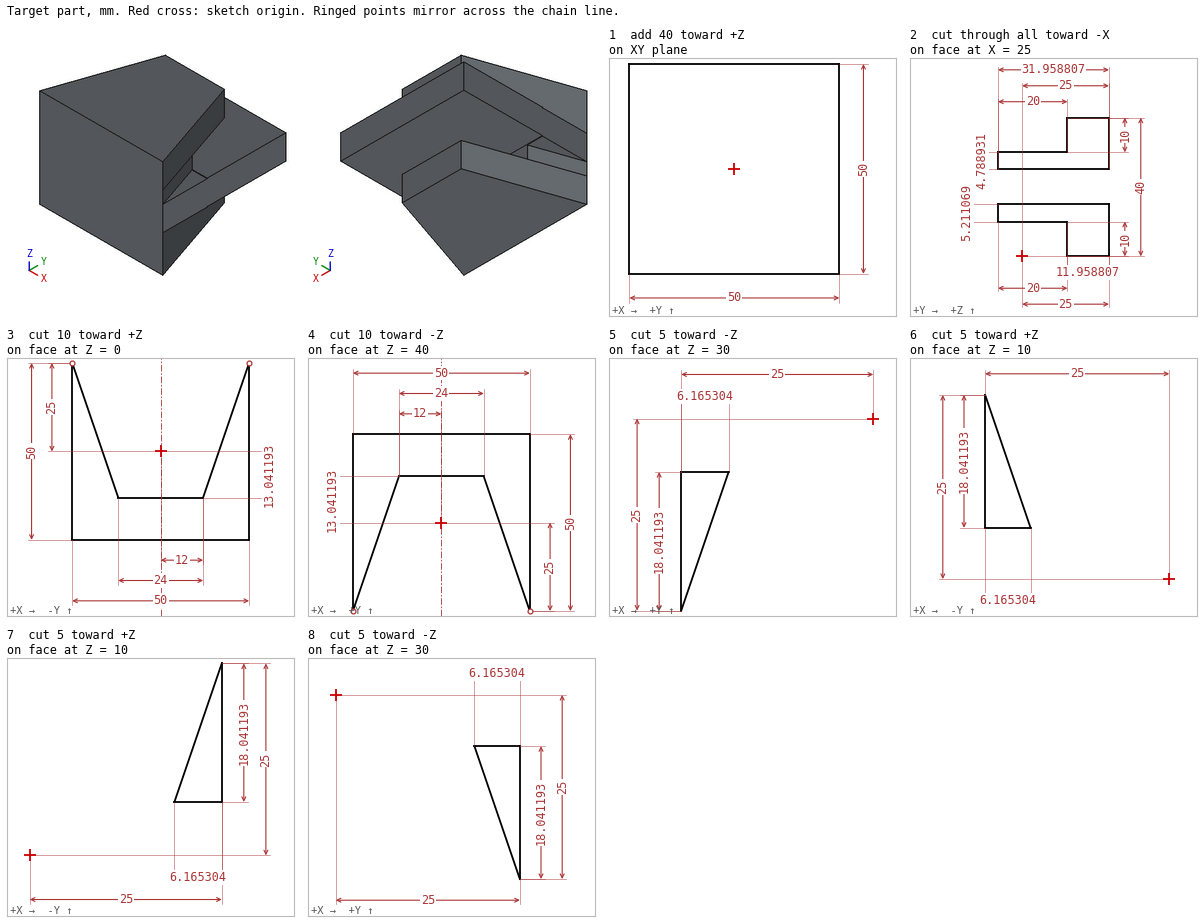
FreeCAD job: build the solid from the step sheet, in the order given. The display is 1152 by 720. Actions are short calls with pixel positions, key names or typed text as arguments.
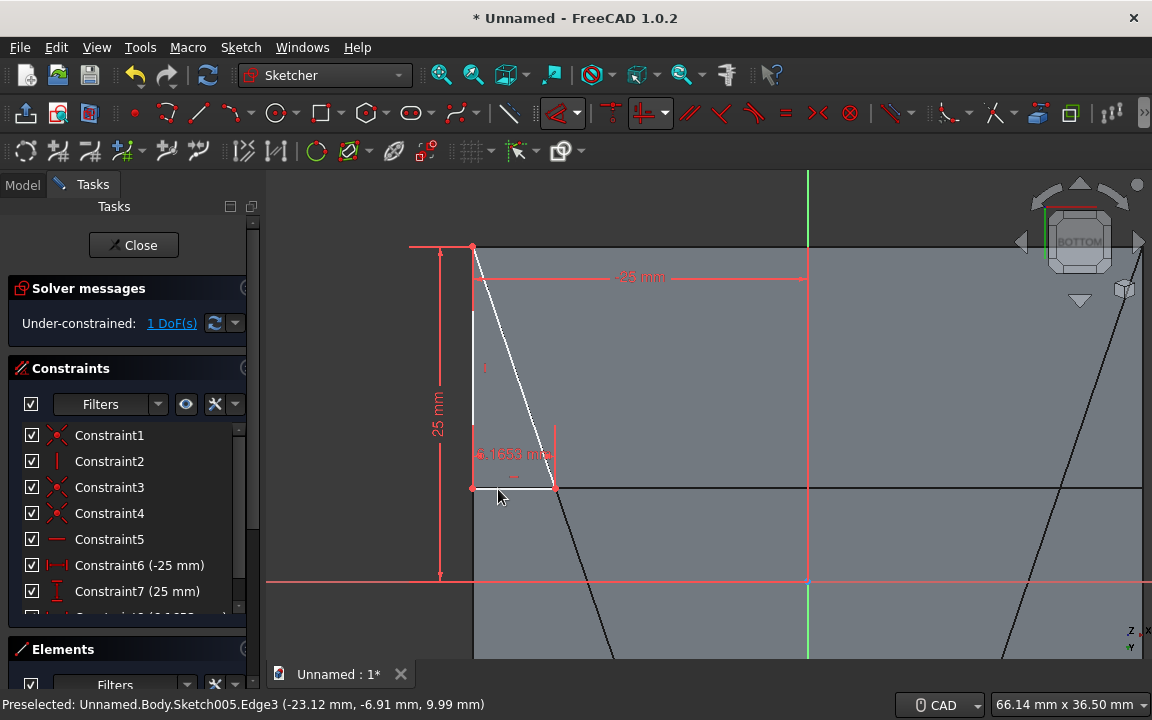
click(473, 319)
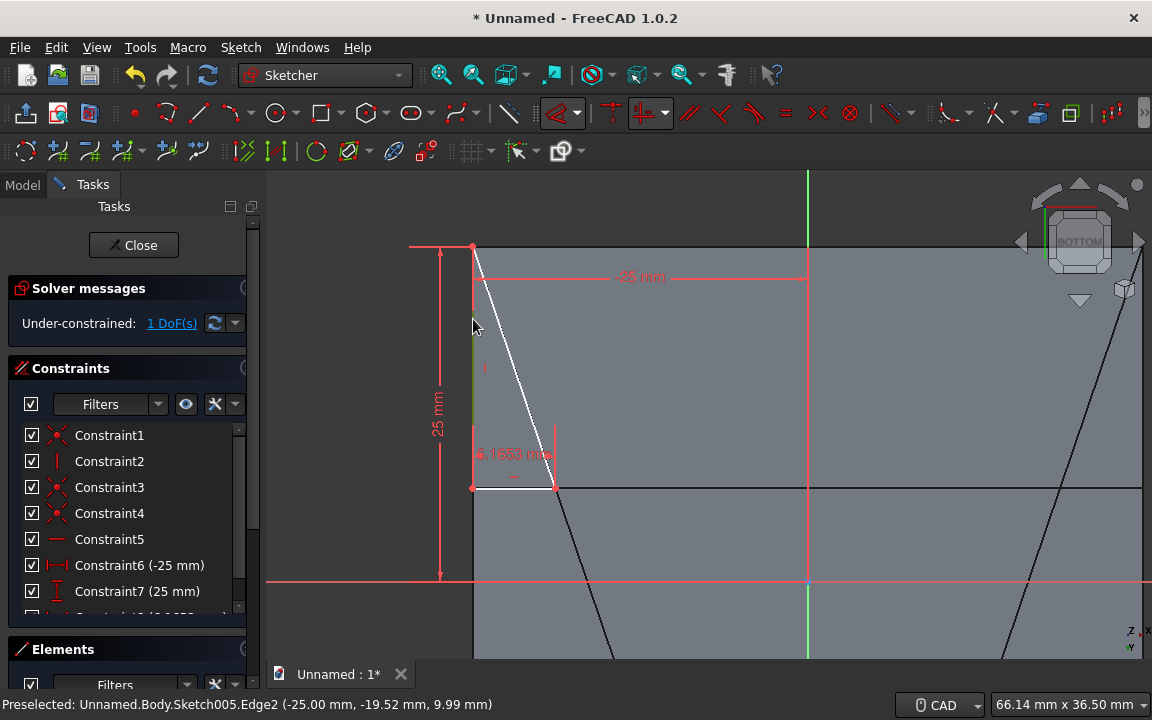
key(i)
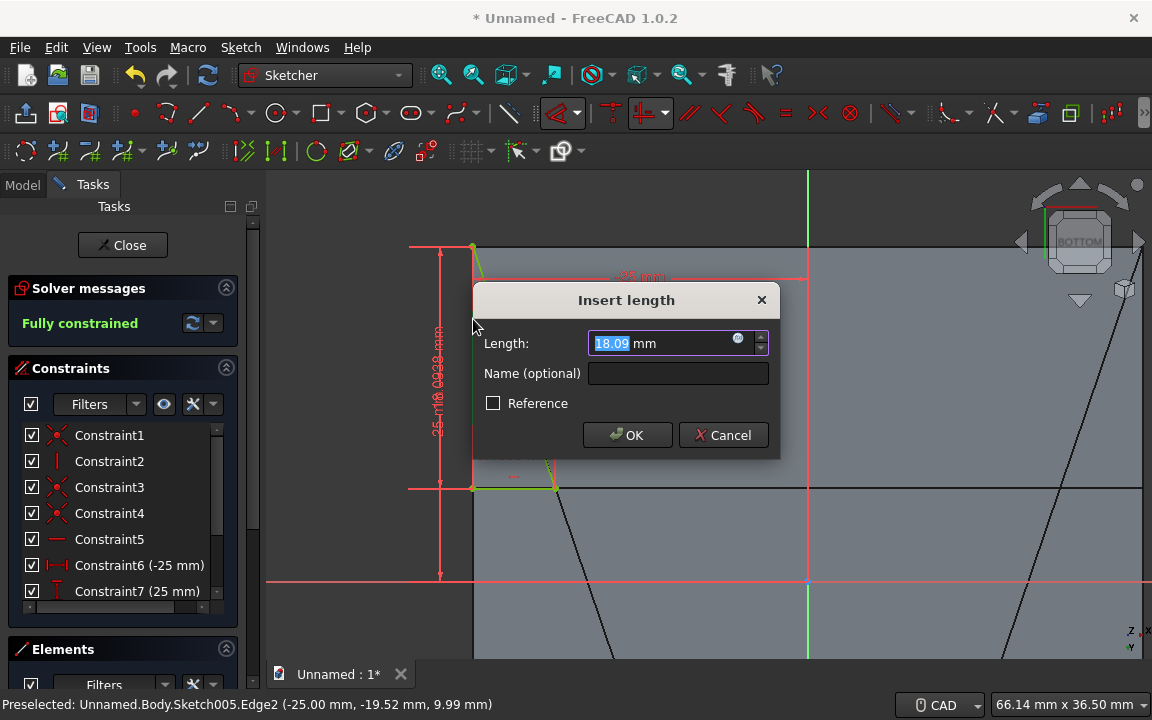
text(18.041193)
key(Return)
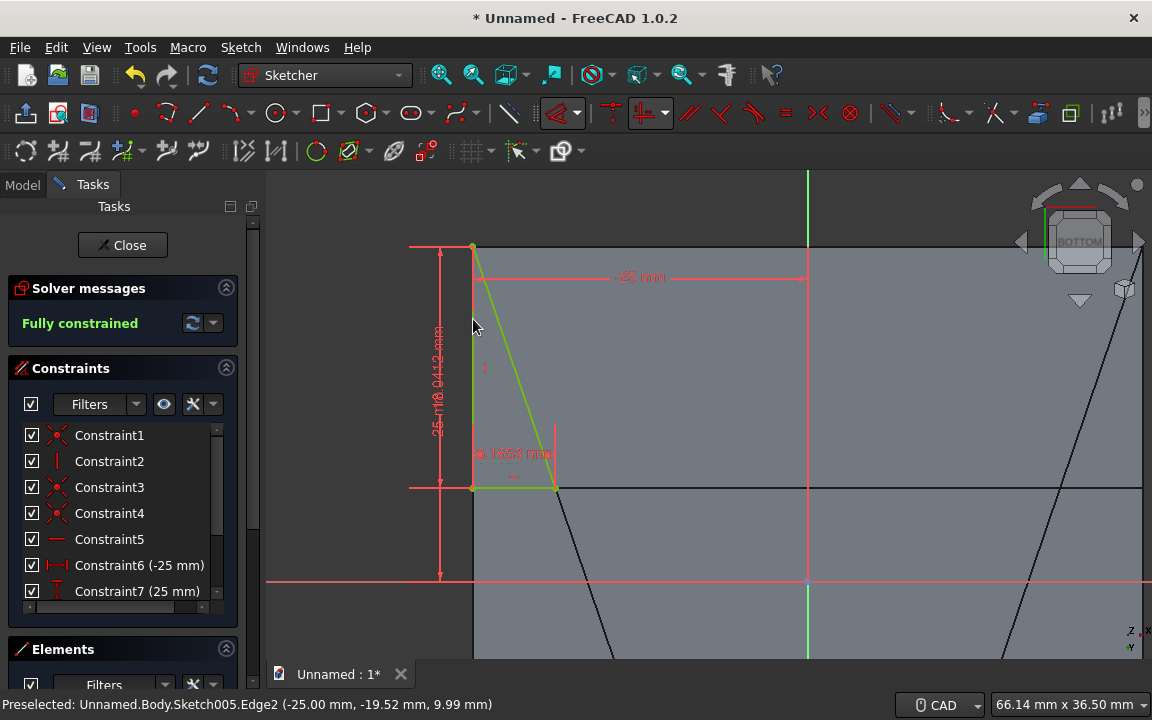
click(123, 245)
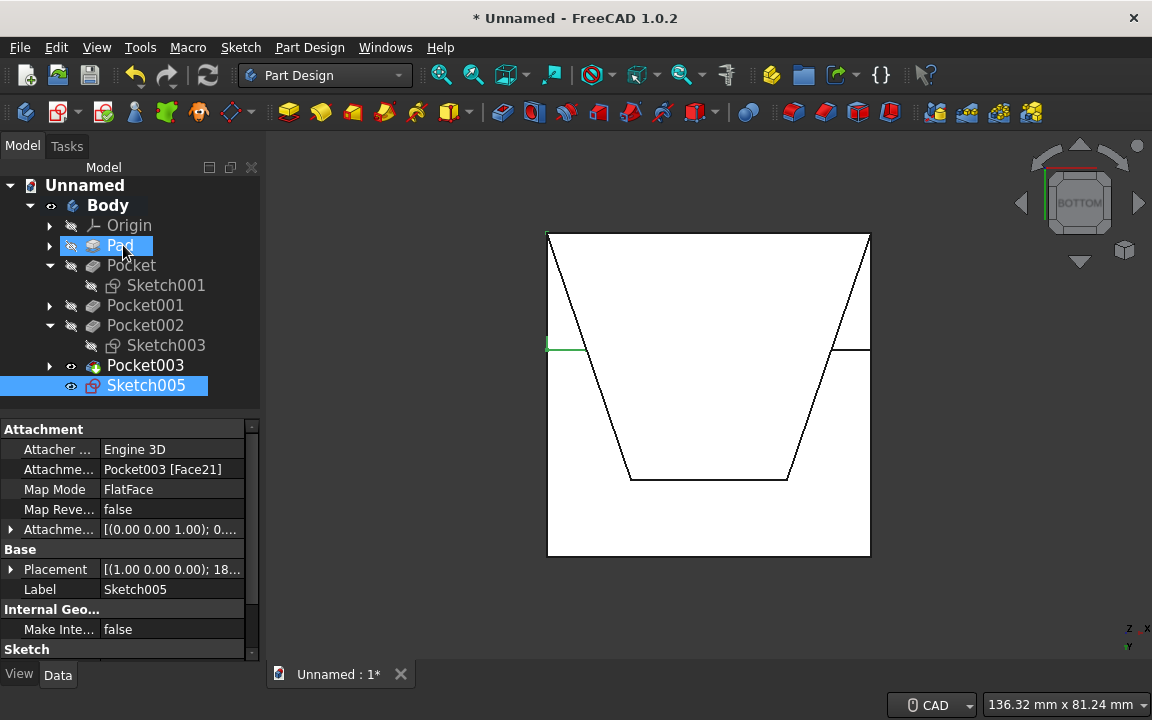
click(504, 112)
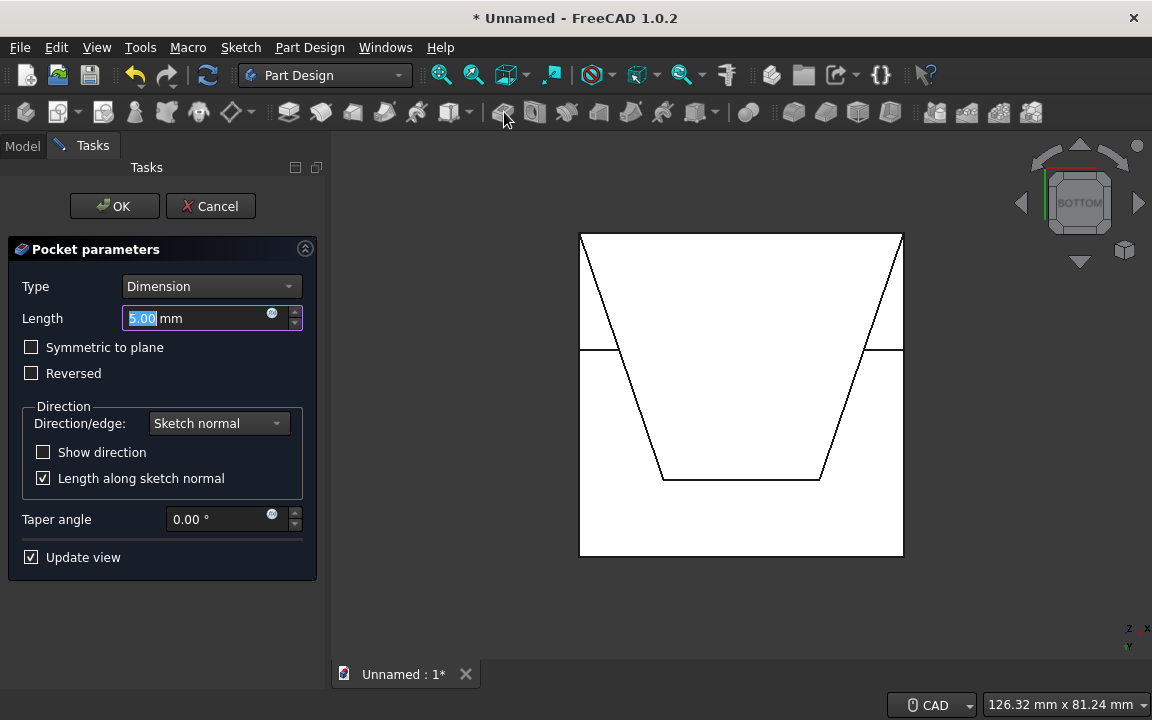
text(5)
key(Tab)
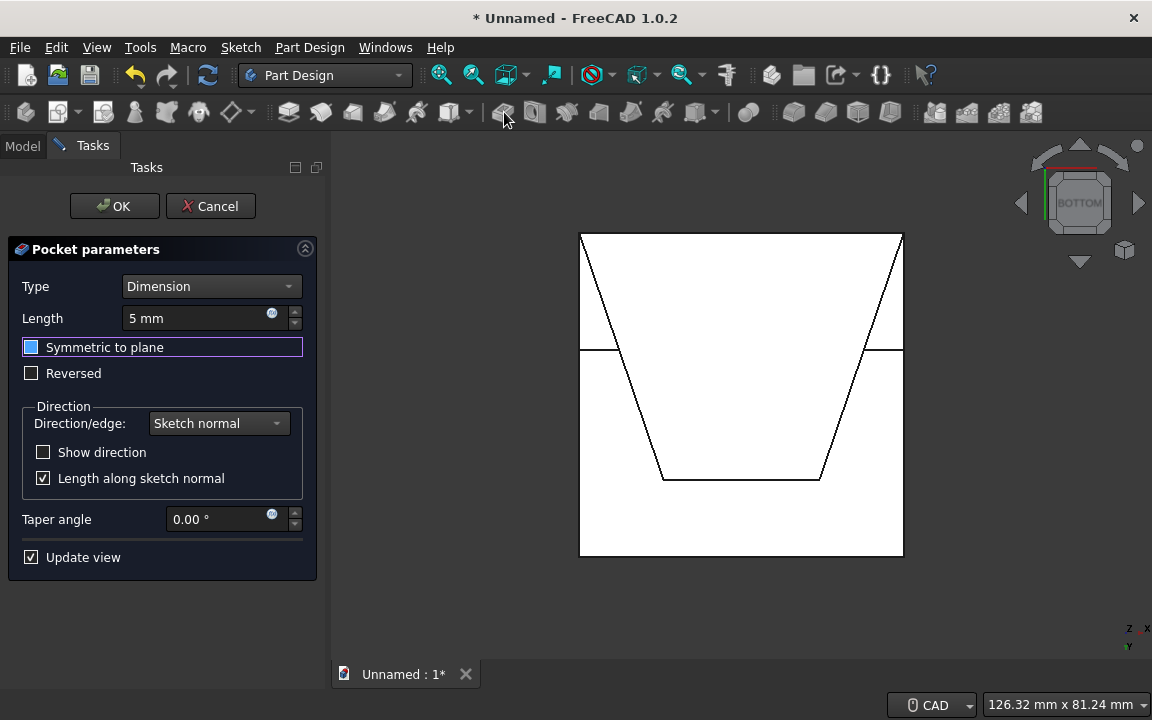
click(115, 206)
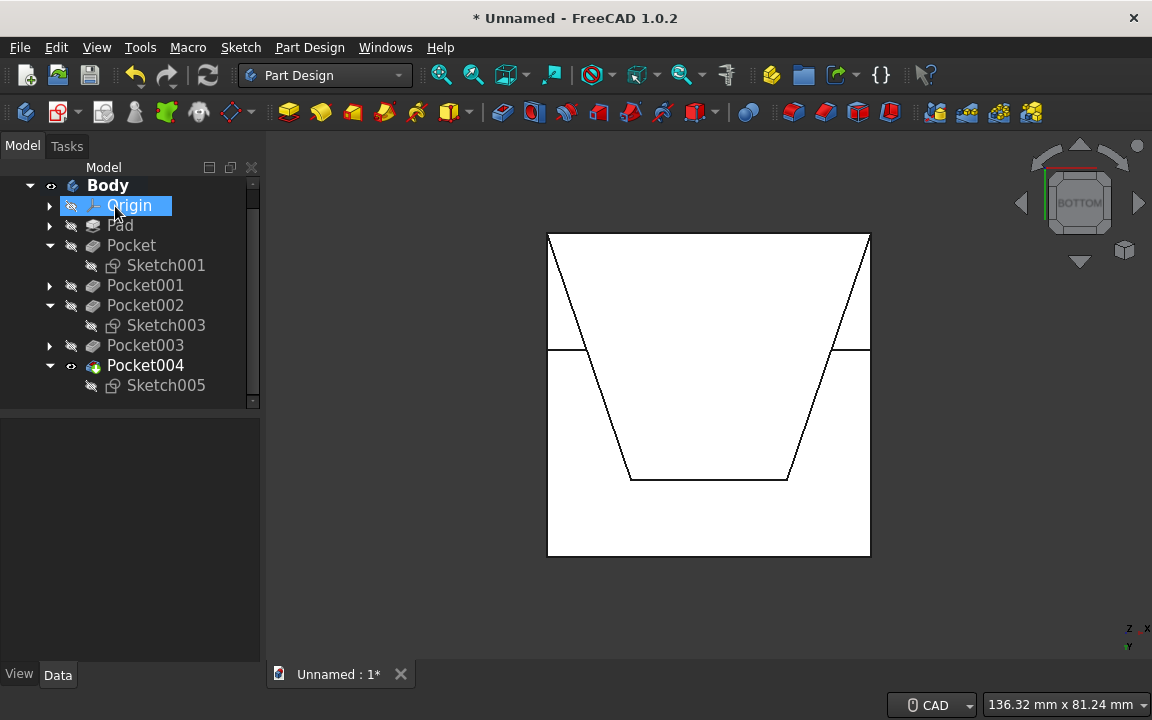
click(857, 324)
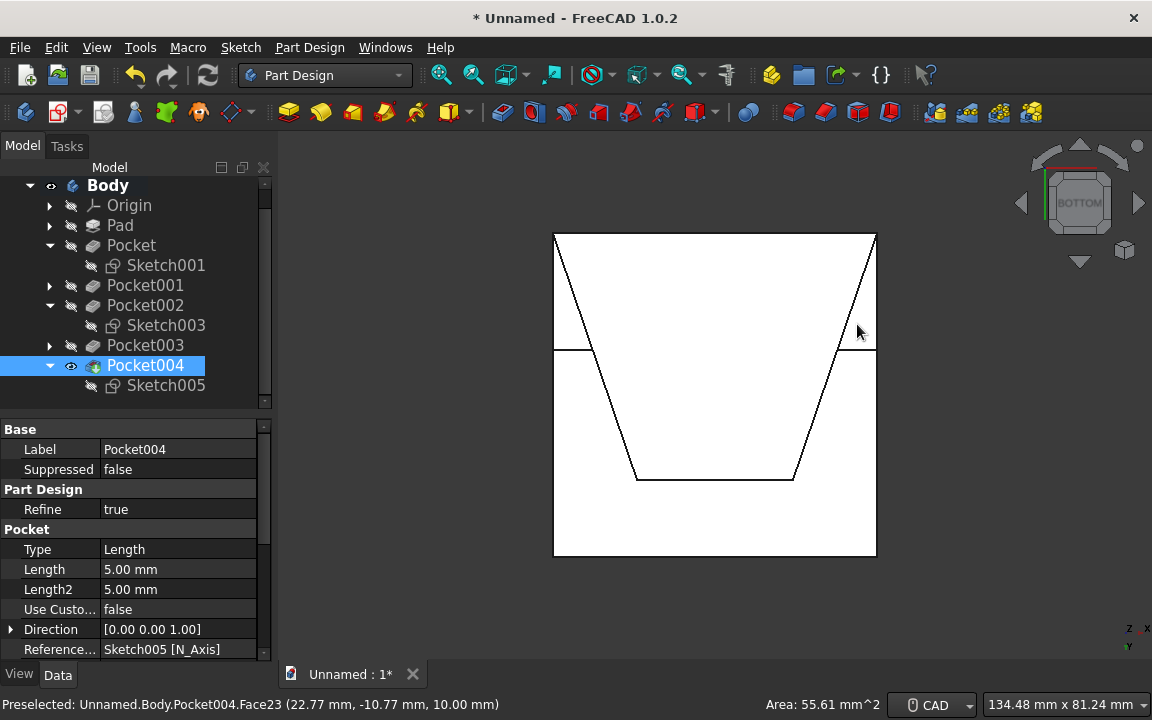
click(58, 112)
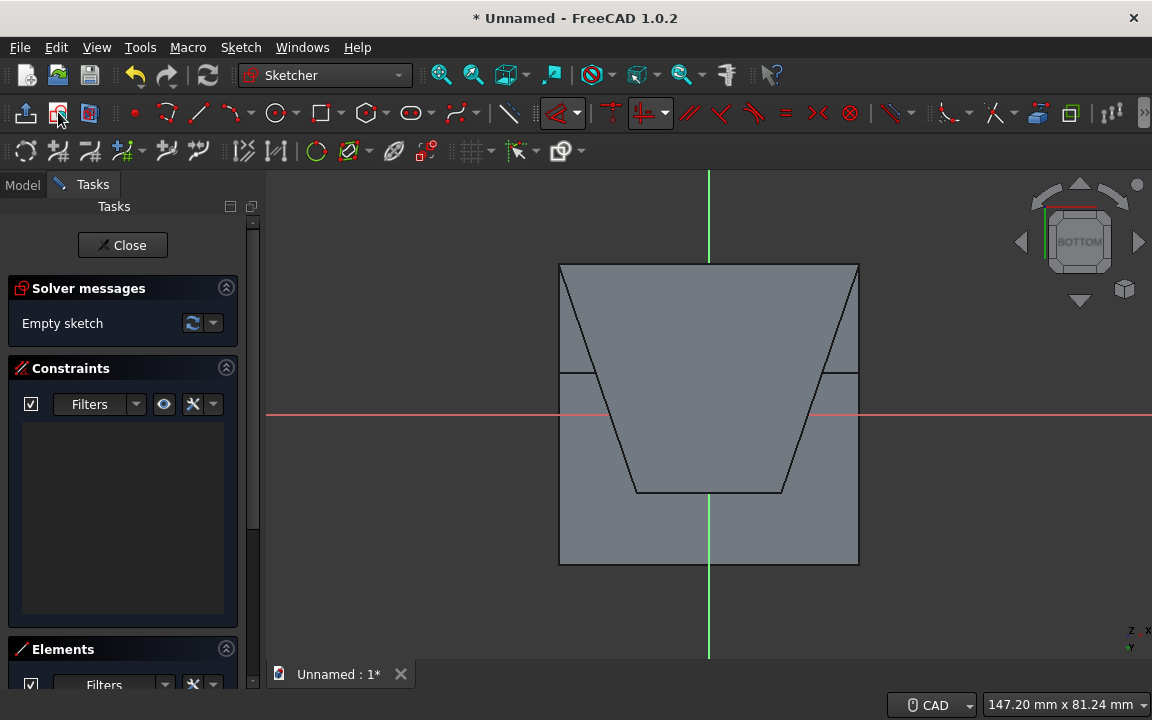
scroll(902, 278, up, 4)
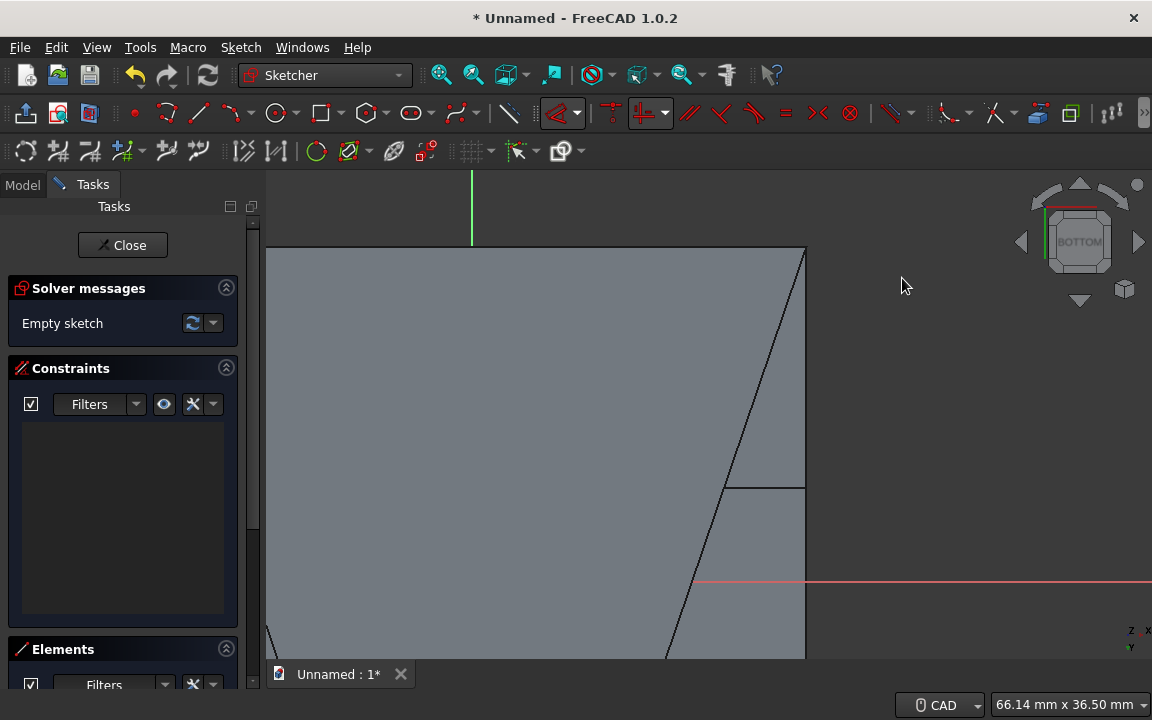
key(g)
key(m)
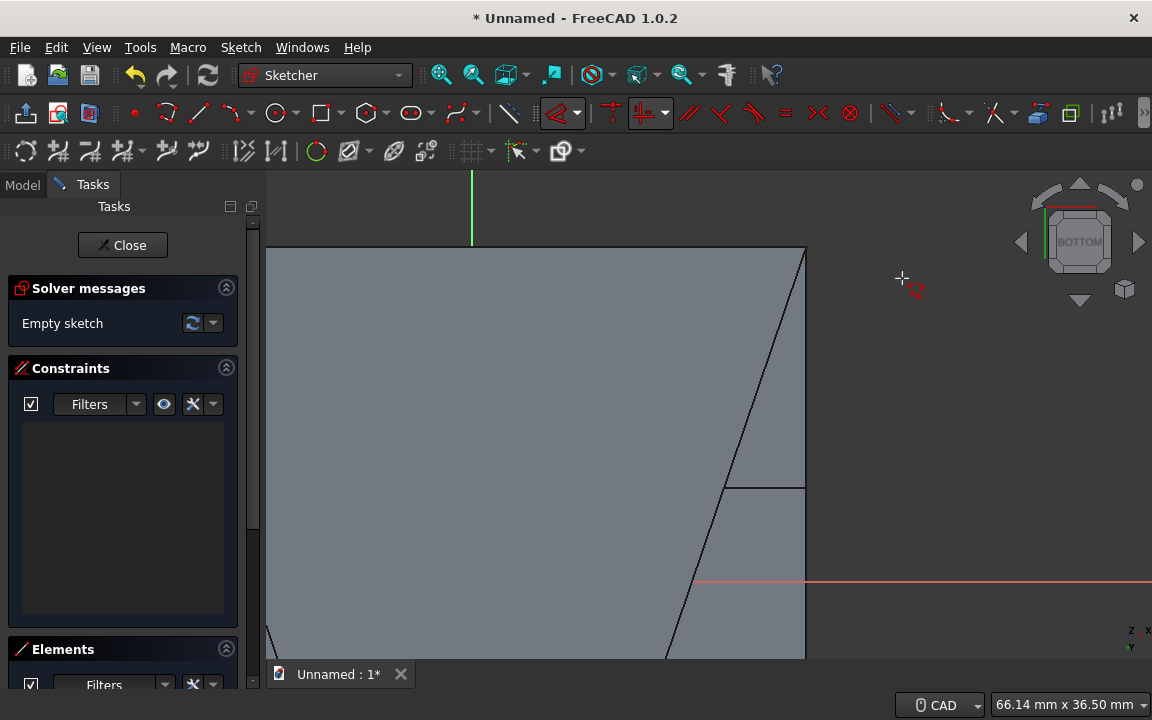
click(724, 488)
click(806, 488)
click(806, 247)
click(724, 489)
key(Escape)
key(Escape)